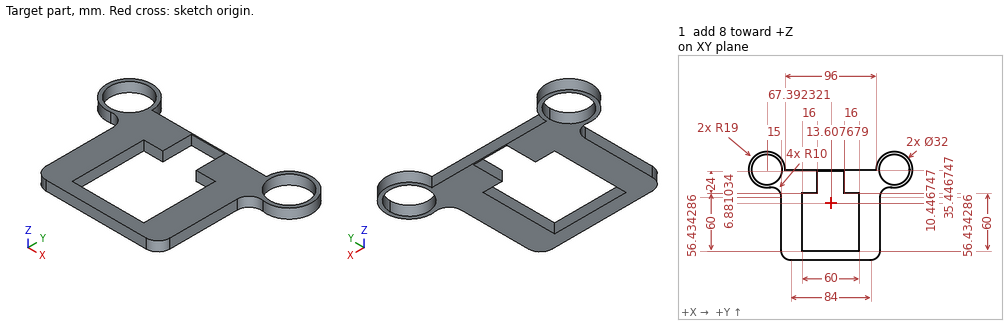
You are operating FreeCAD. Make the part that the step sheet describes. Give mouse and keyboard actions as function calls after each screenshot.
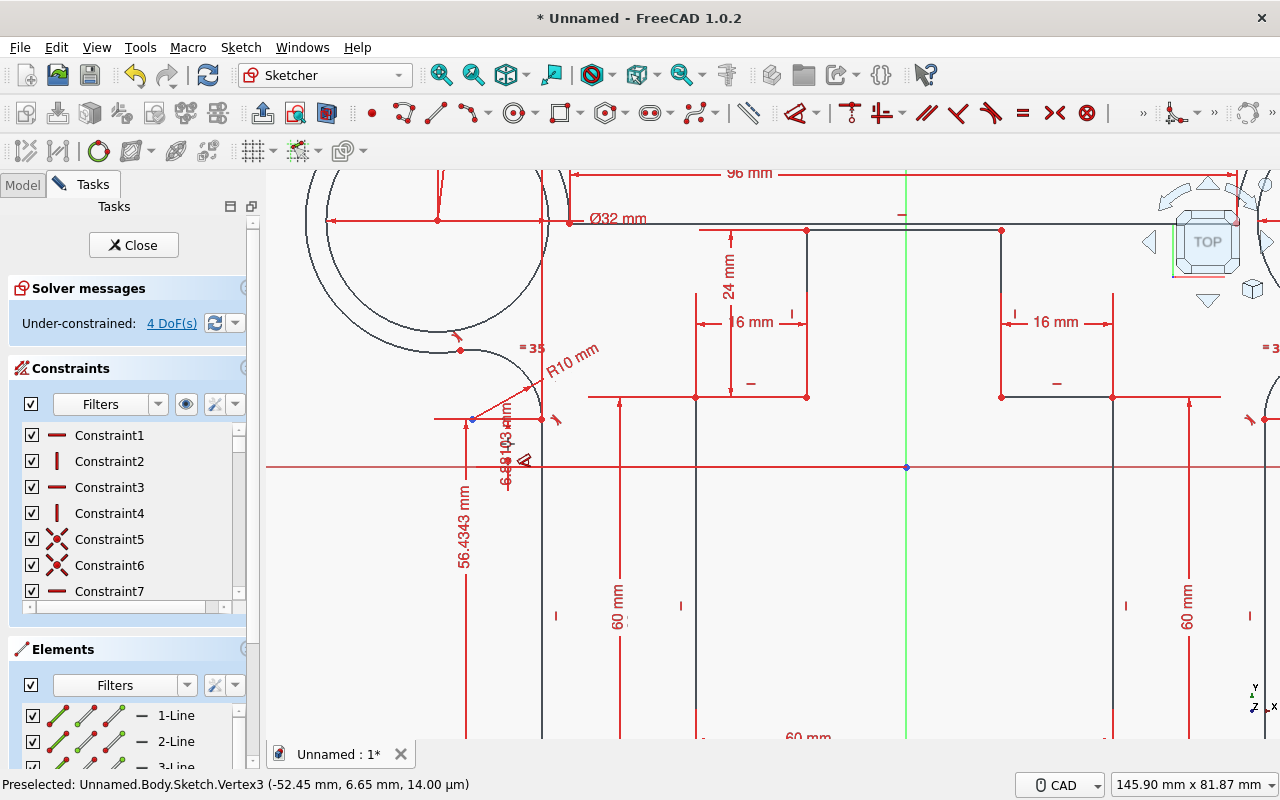
click(438, 221)
click(672, 501)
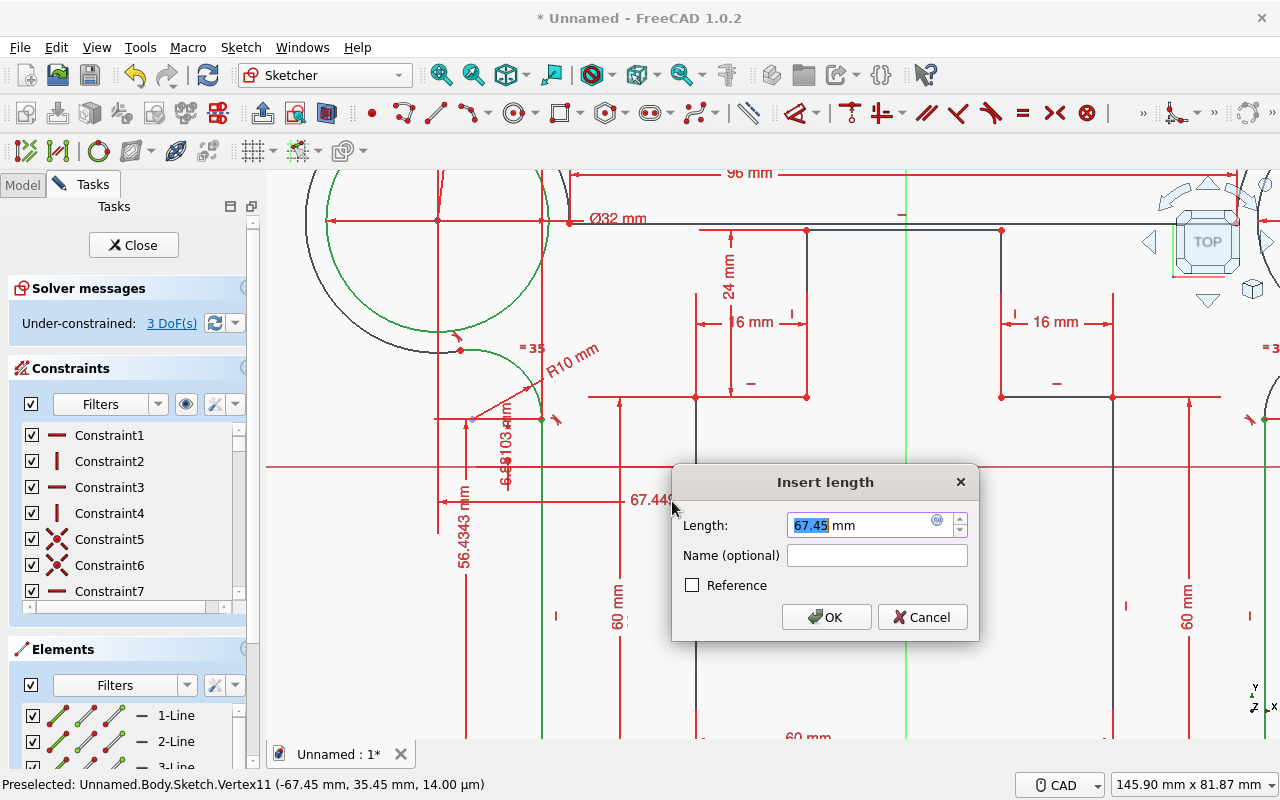
text(67.392321)
key(Return)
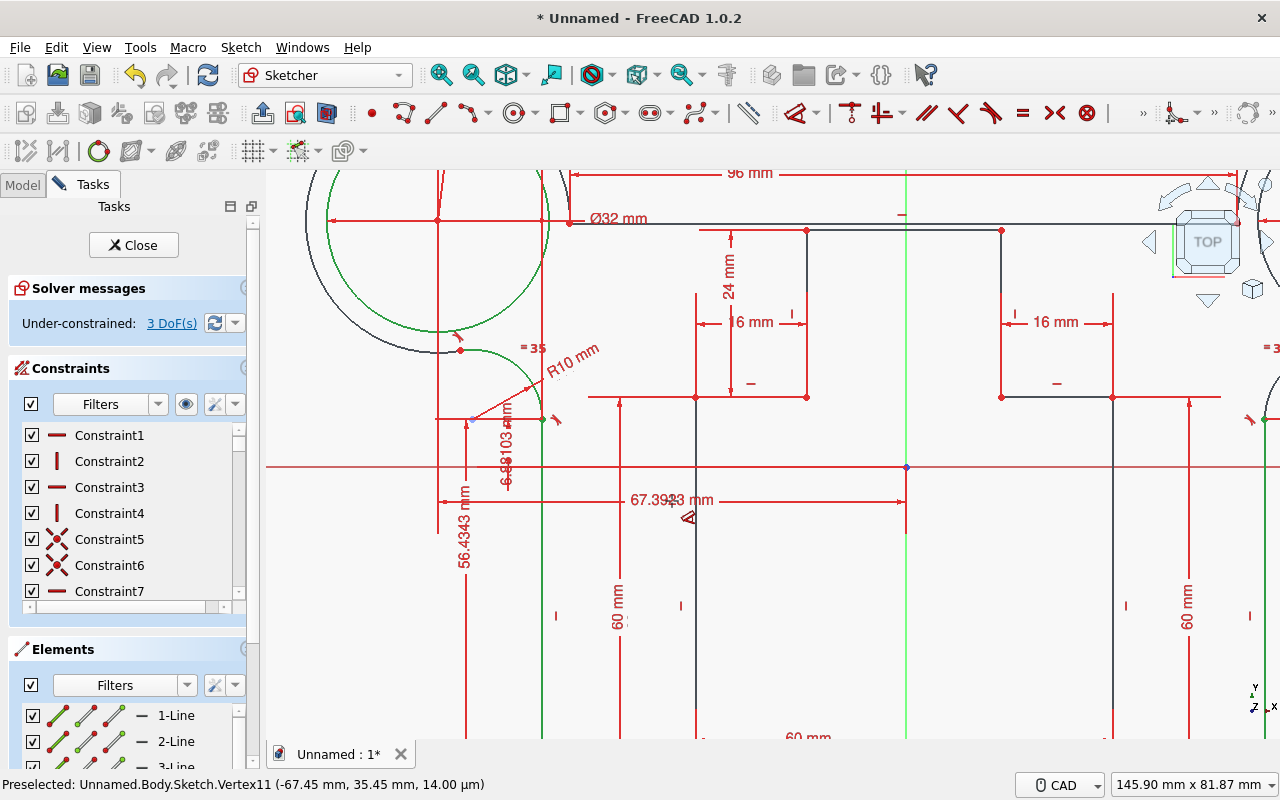
scroll(542, 421, down, 4)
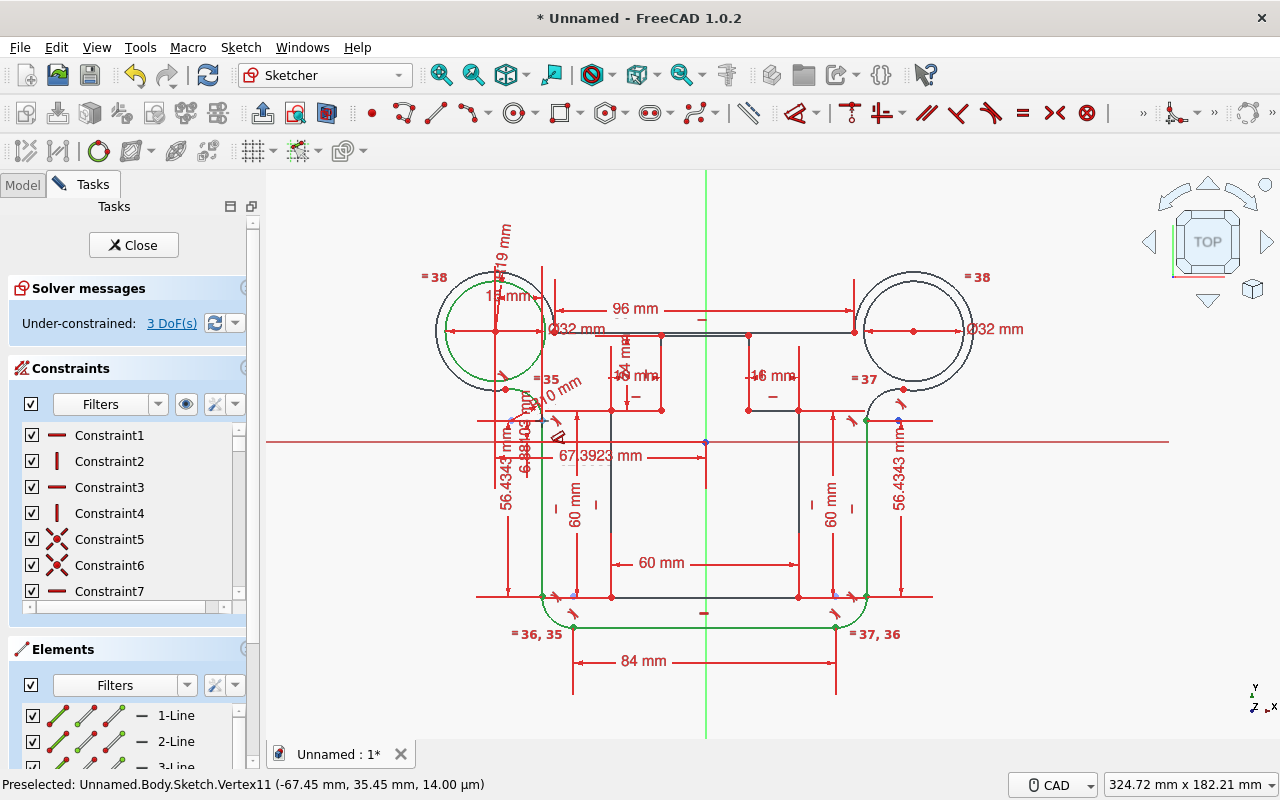
click(854, 333)
click(888, 412)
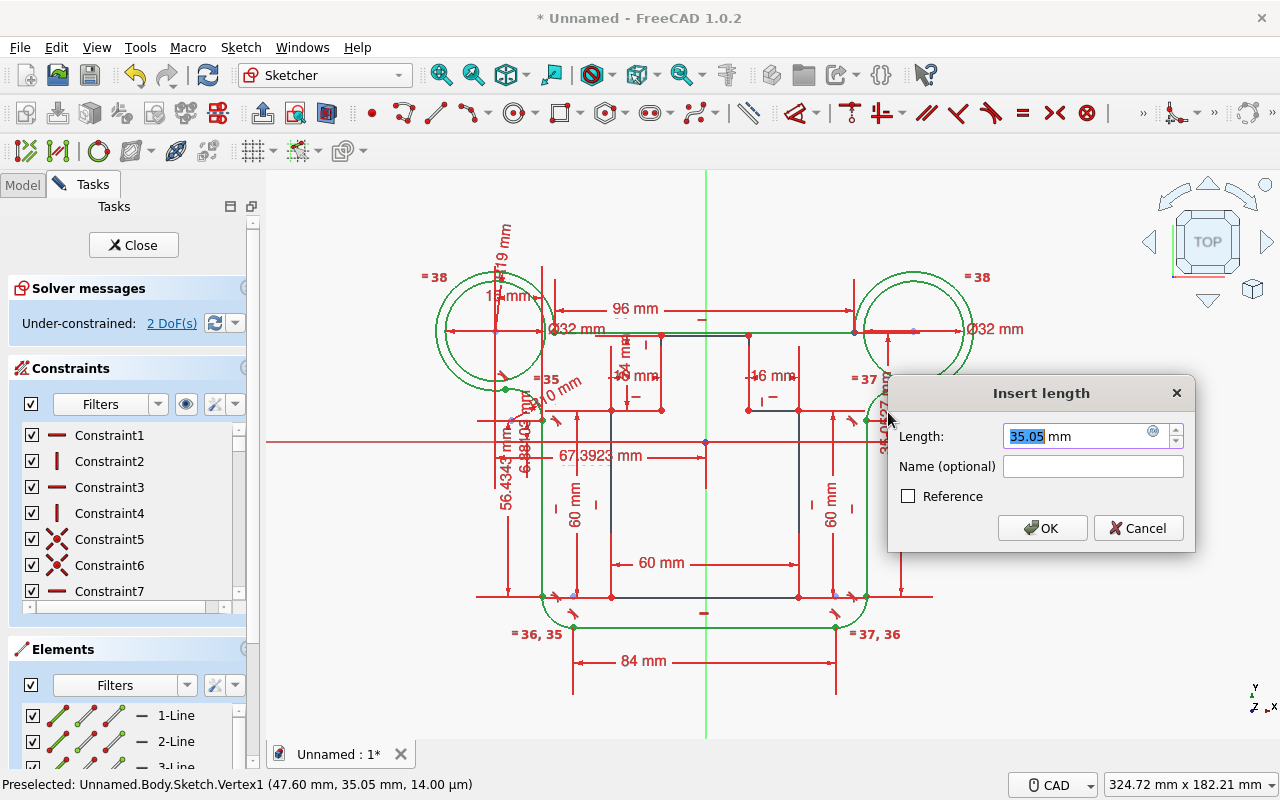
text(35.446747)
key(Return)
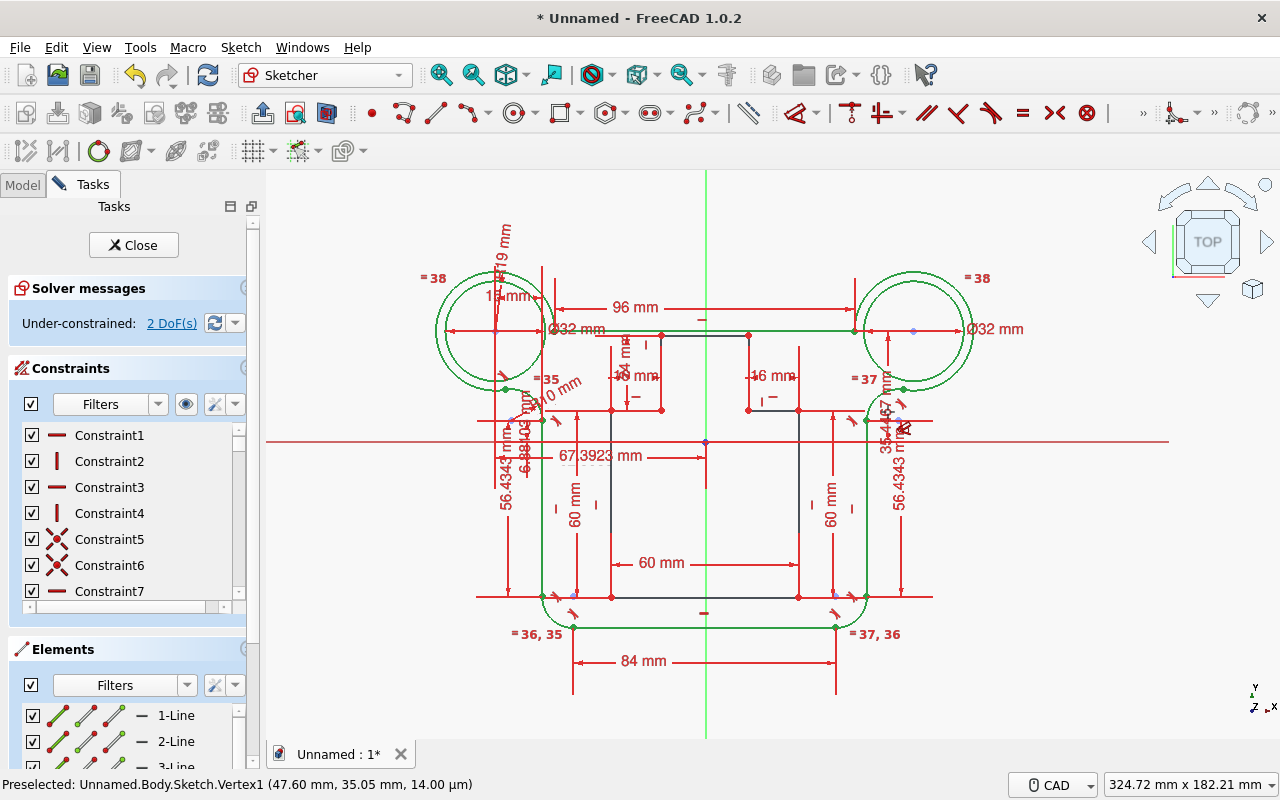
click(749, 411)
click(727, 476)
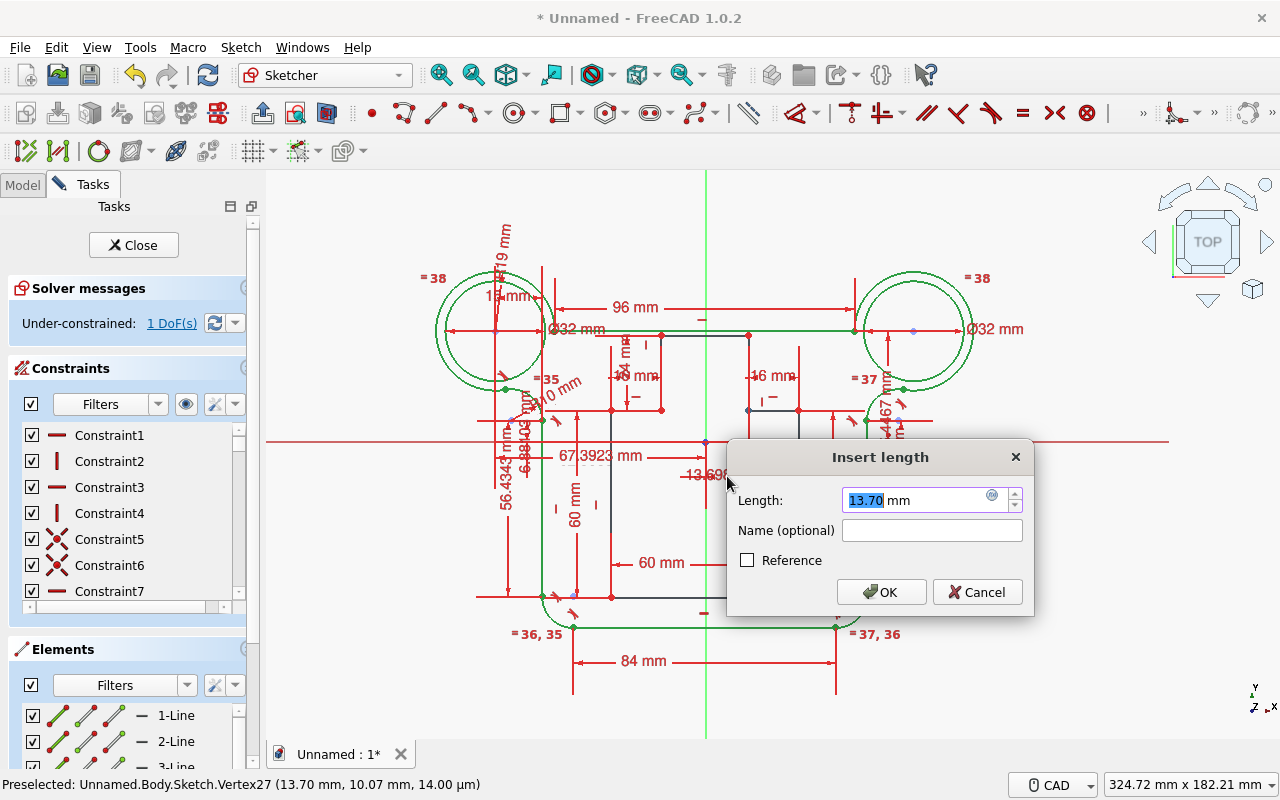
text(13.607679)
key(Return)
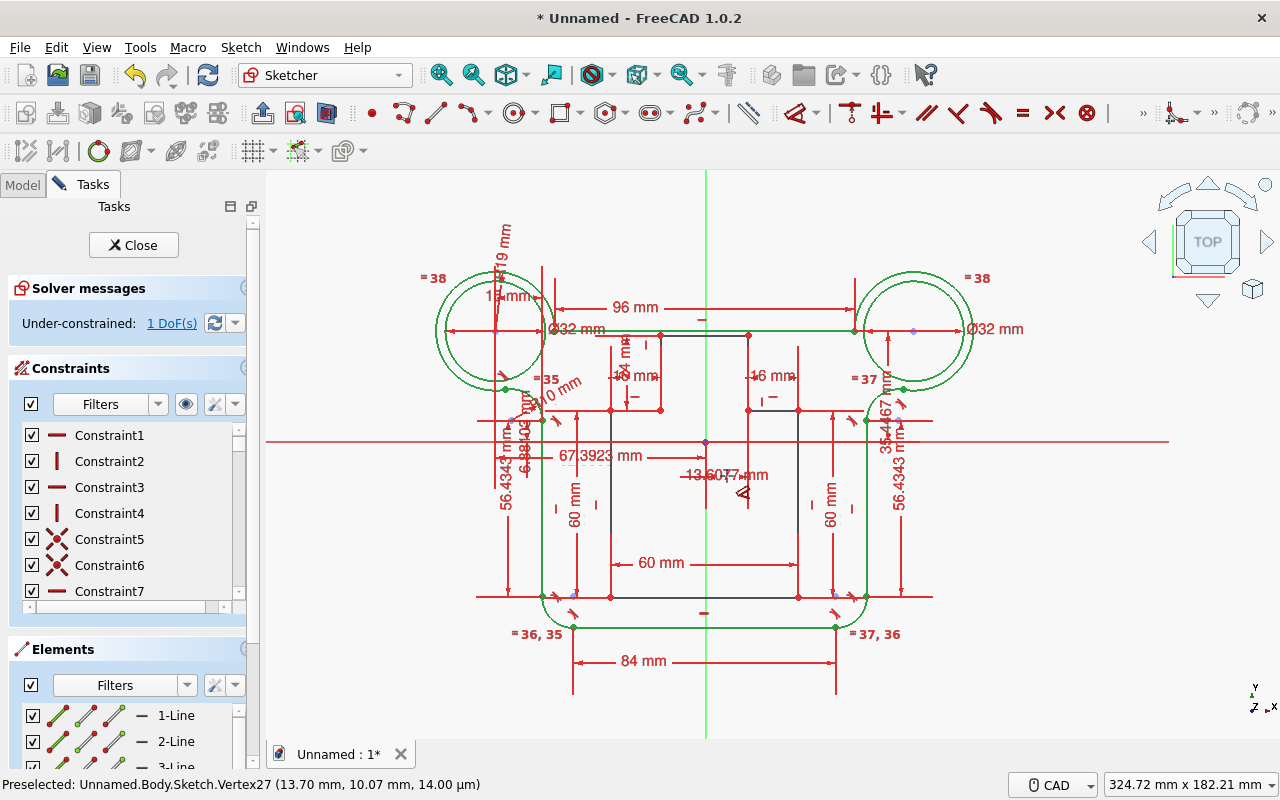
click(748, 411)
click(782, 426)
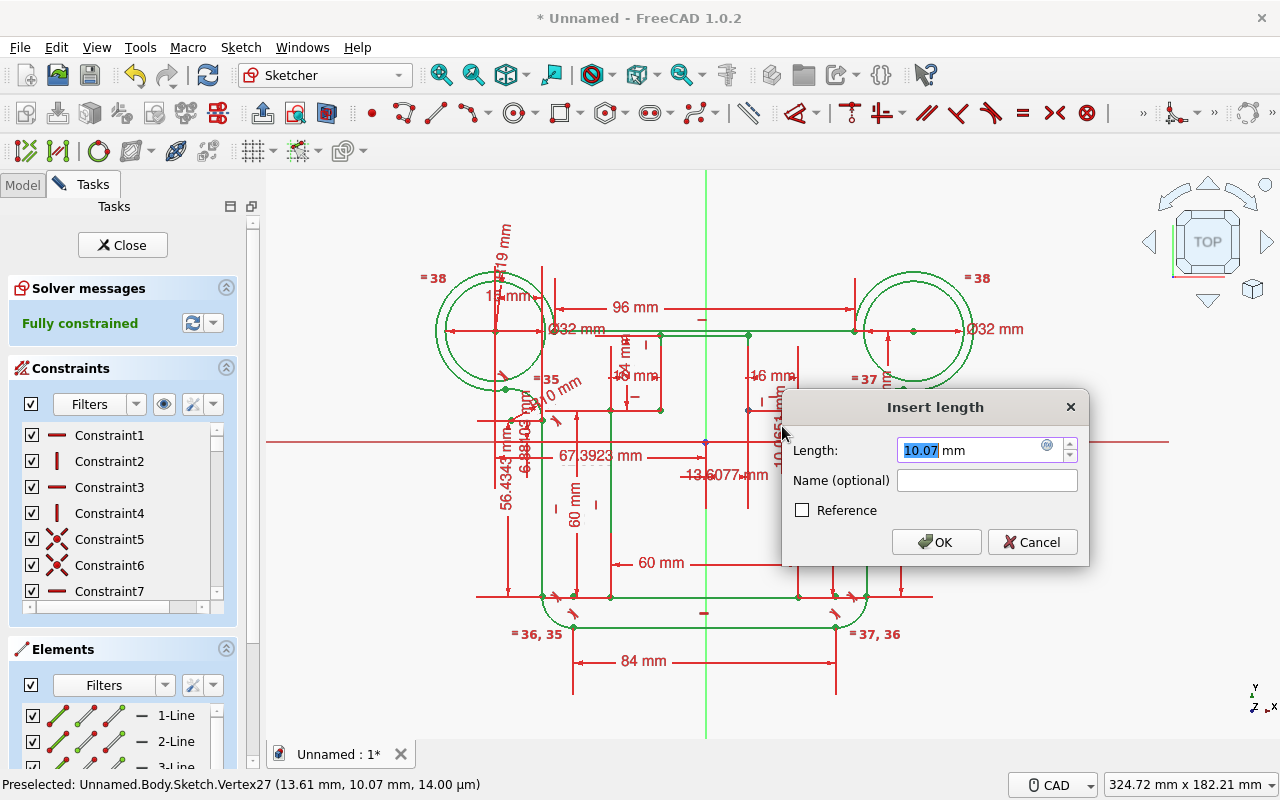
text(10.446747)
key(Return)
key(Escape)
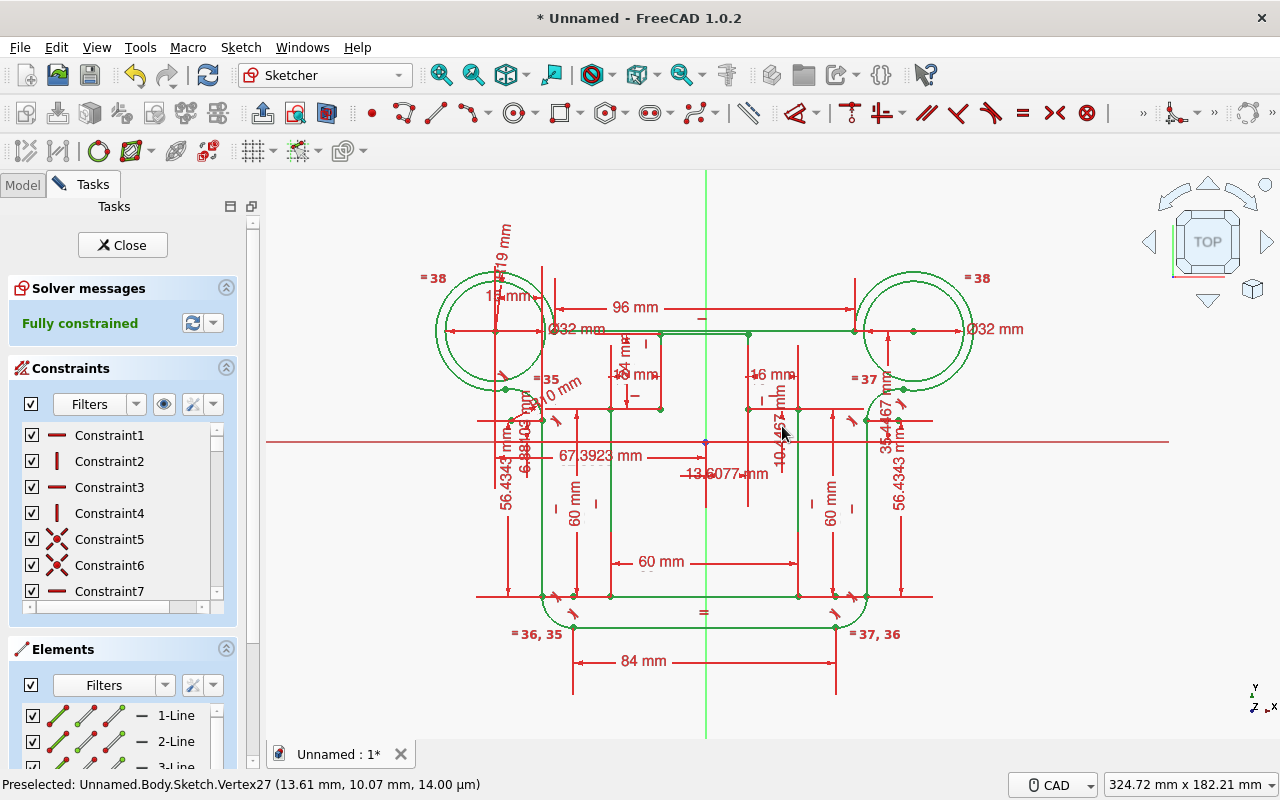
click(123, 245)